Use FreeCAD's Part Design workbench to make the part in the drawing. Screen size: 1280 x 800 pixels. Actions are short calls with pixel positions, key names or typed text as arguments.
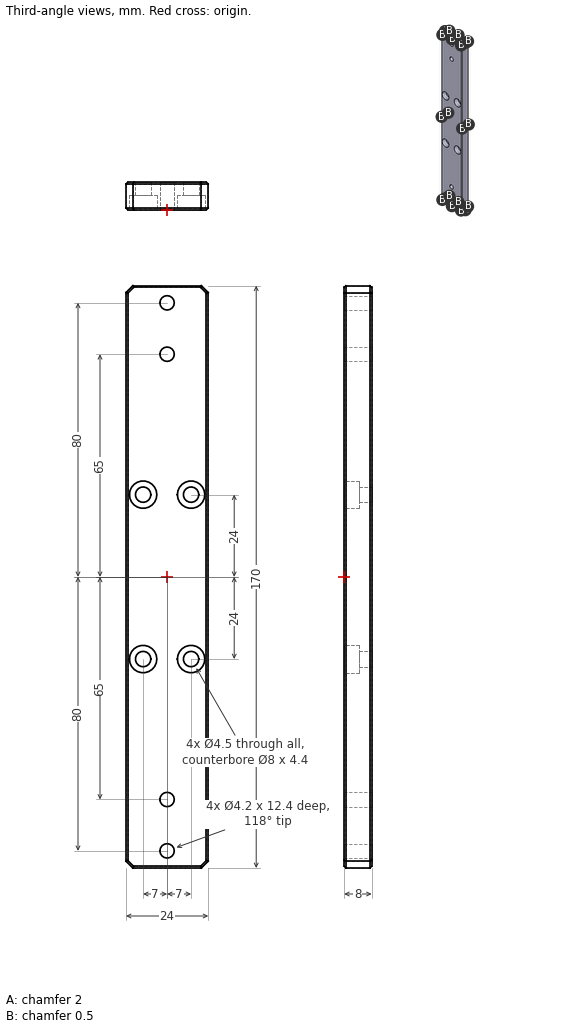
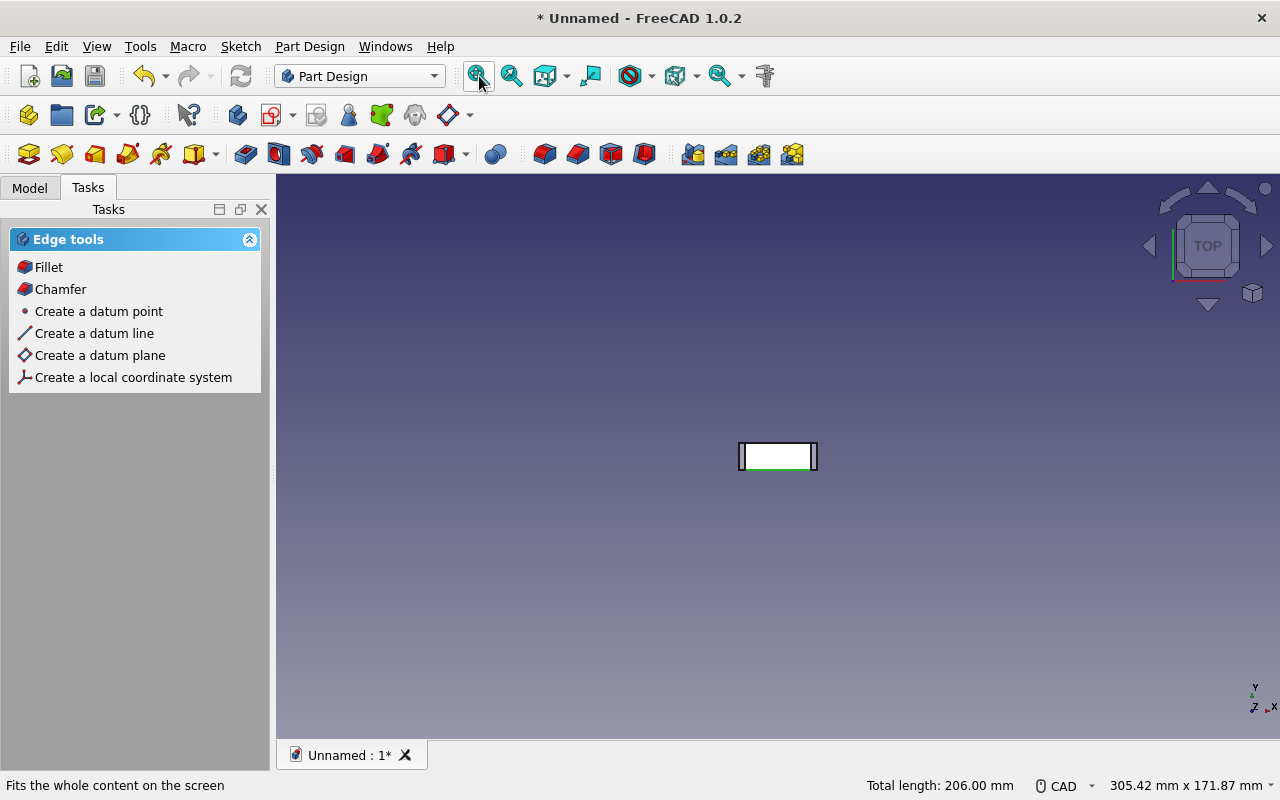
click(778, 442, ctrl)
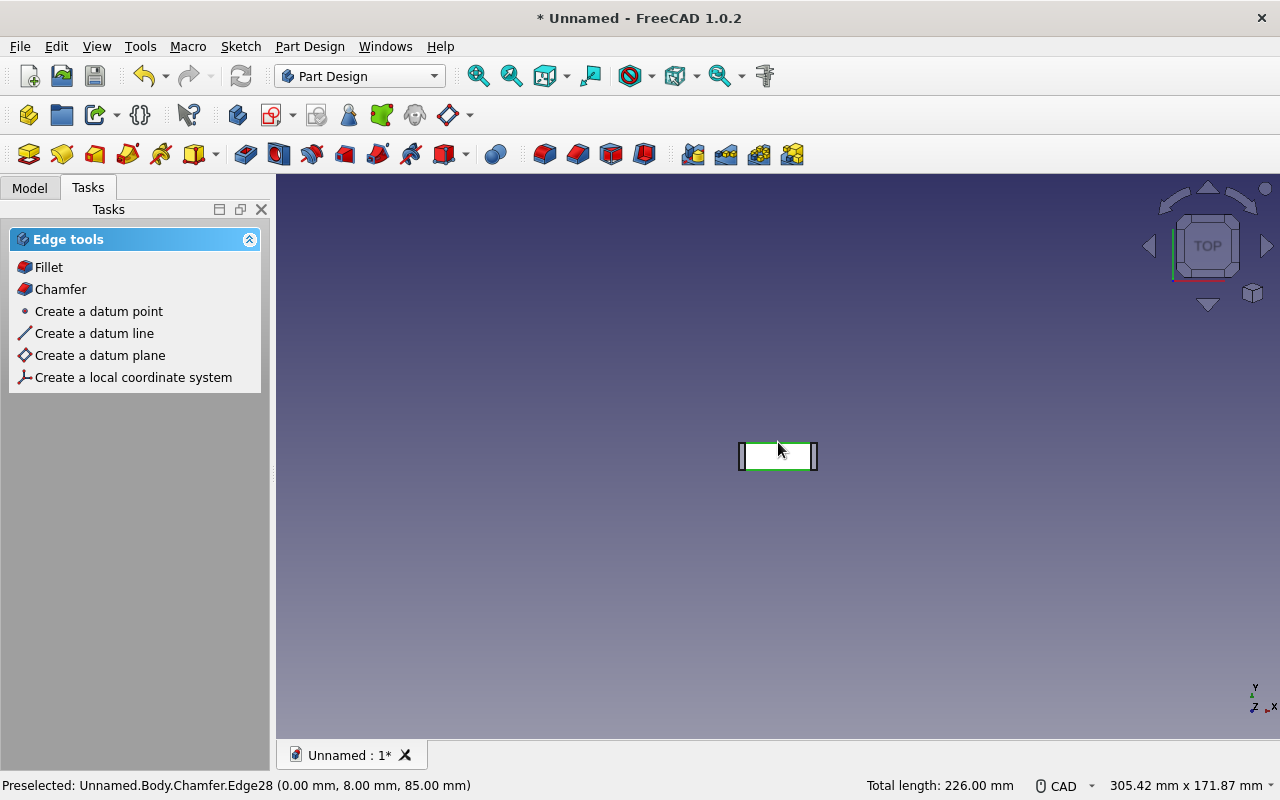
key(1)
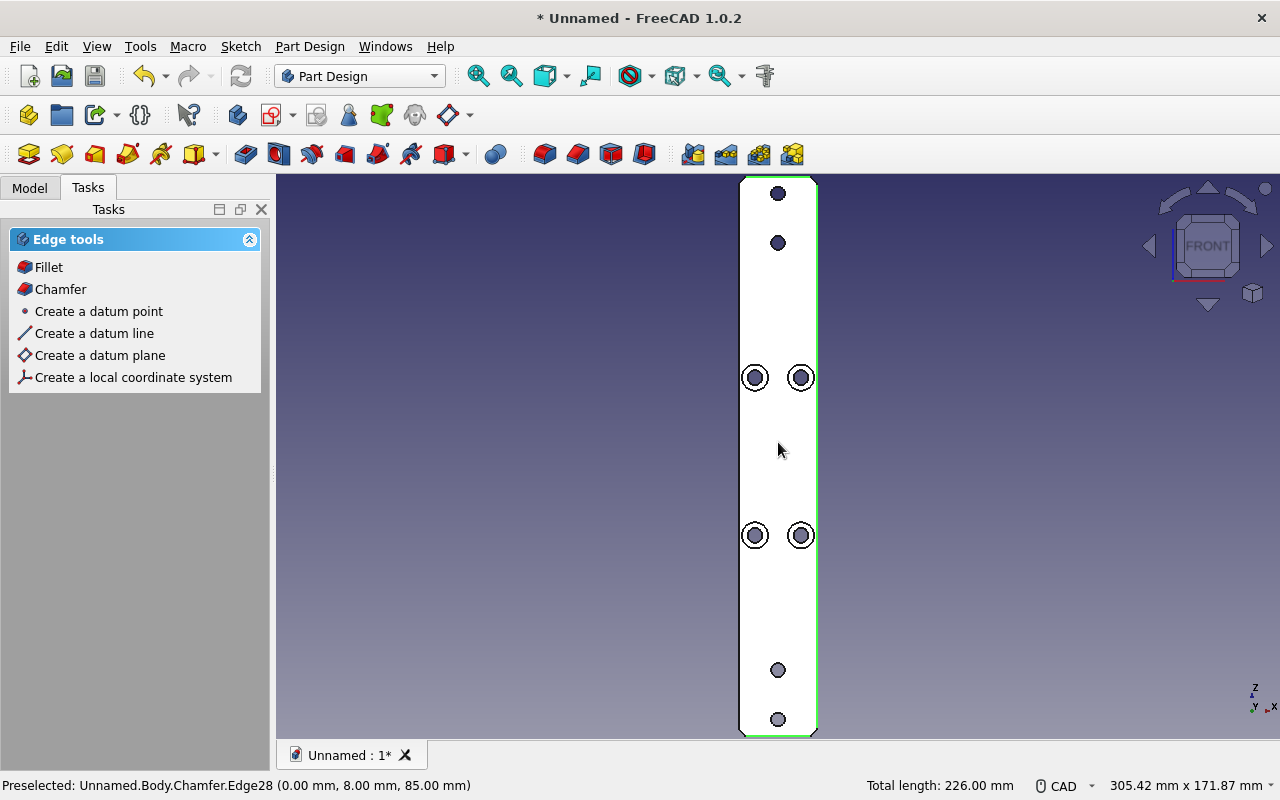
click(739, 456, ctrl)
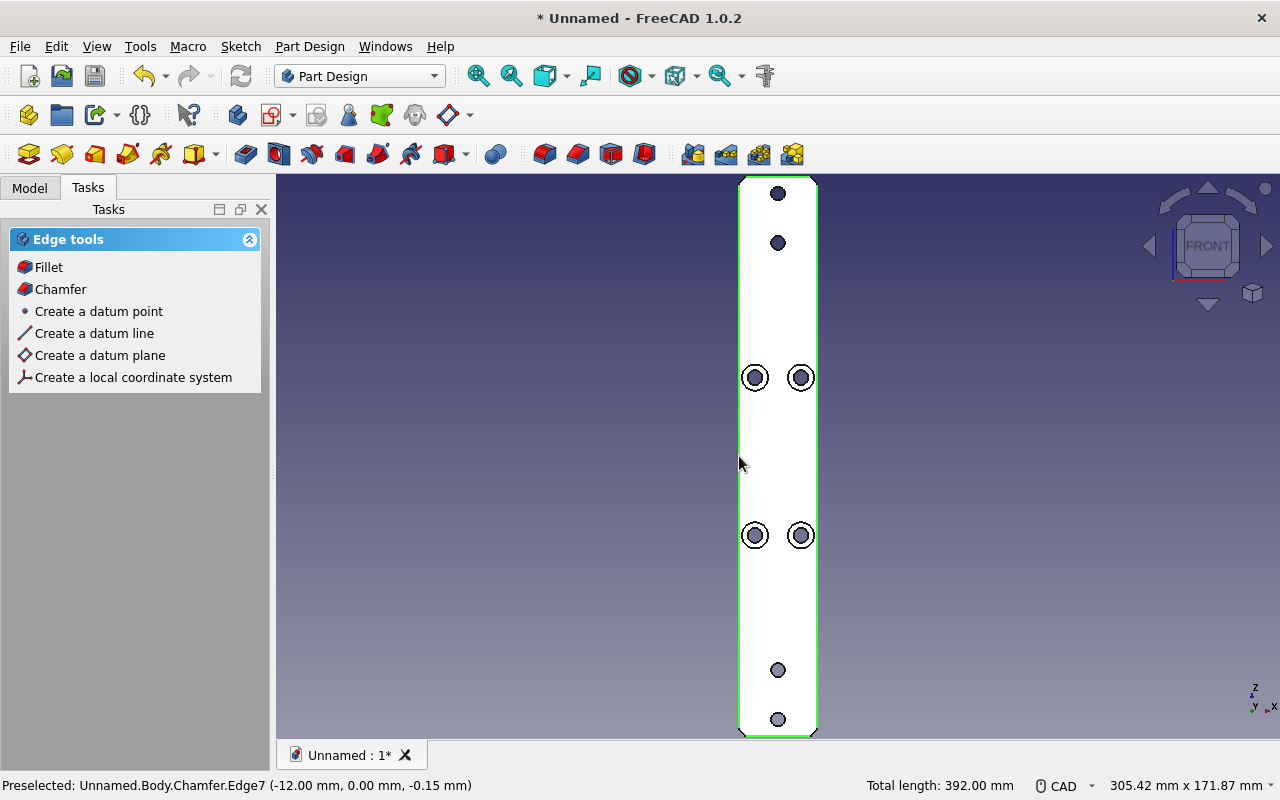
key(3)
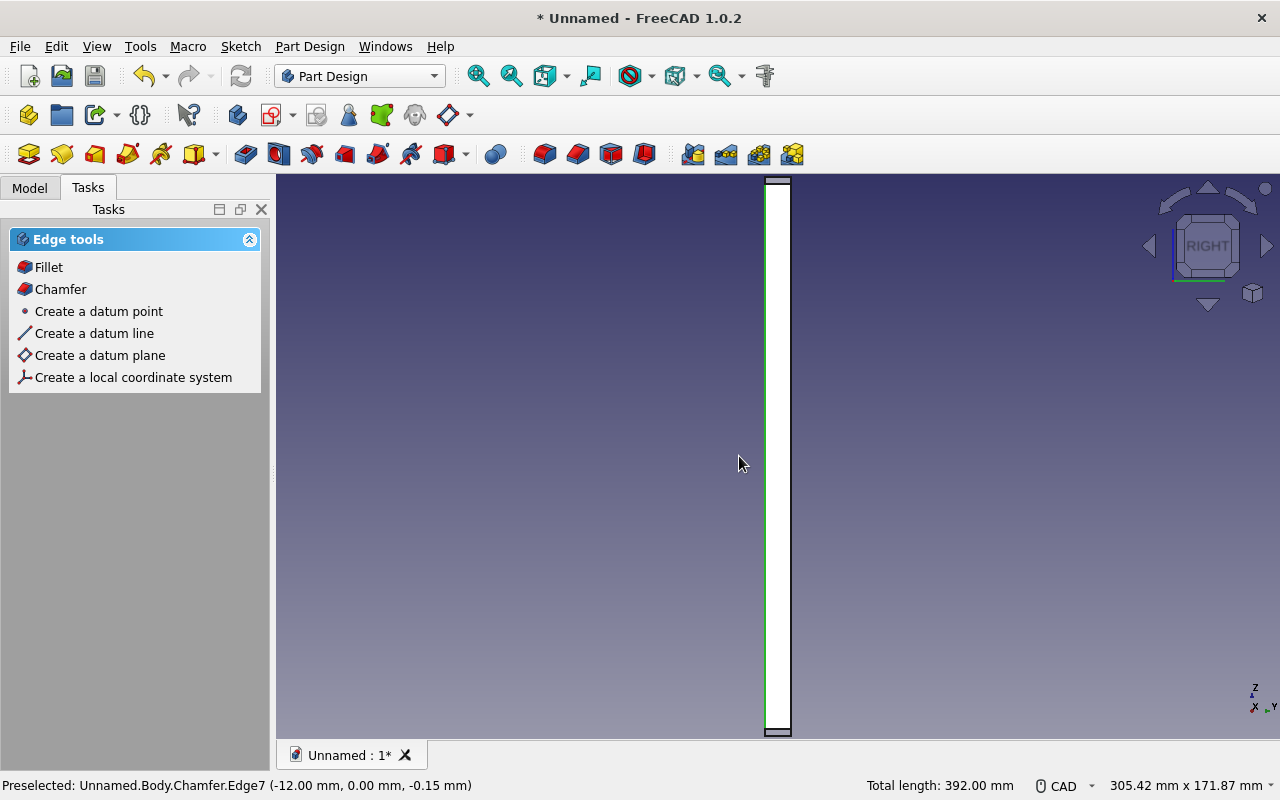
click(791, 455, ctrl)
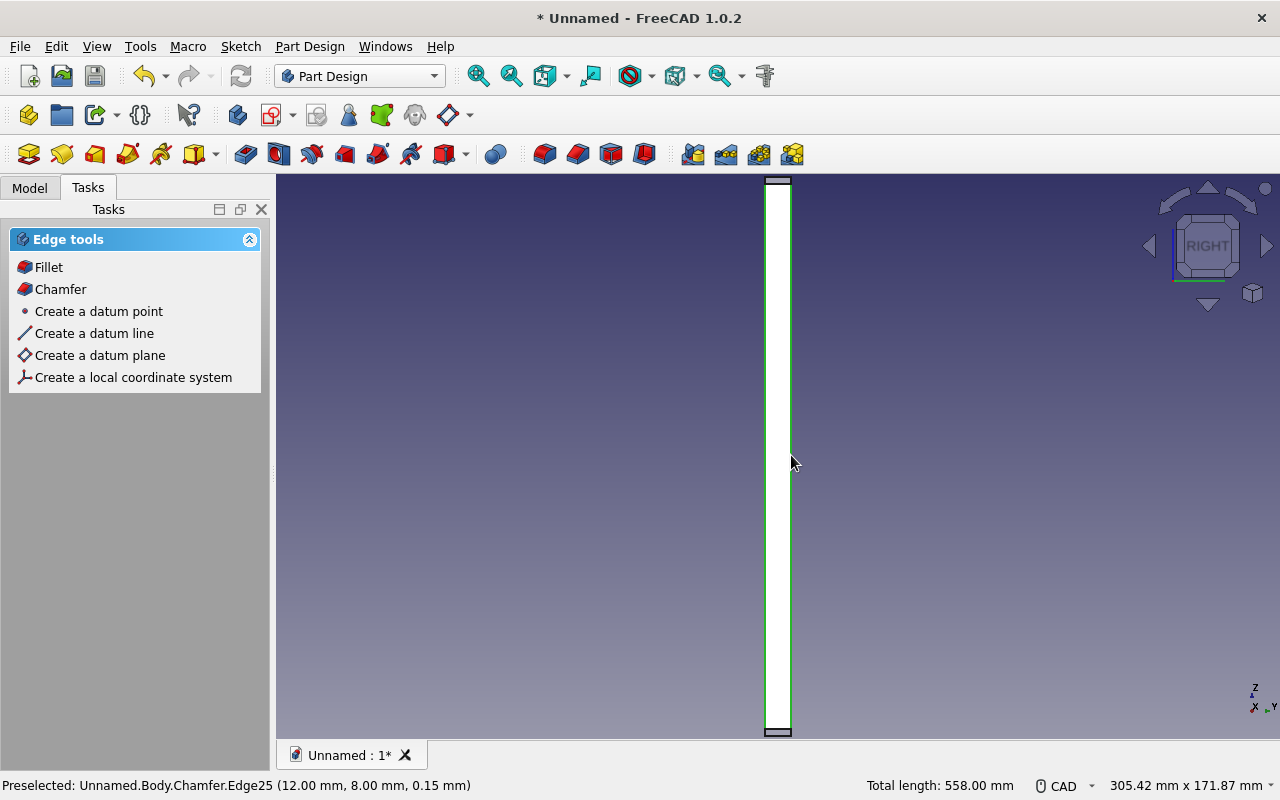
key(5)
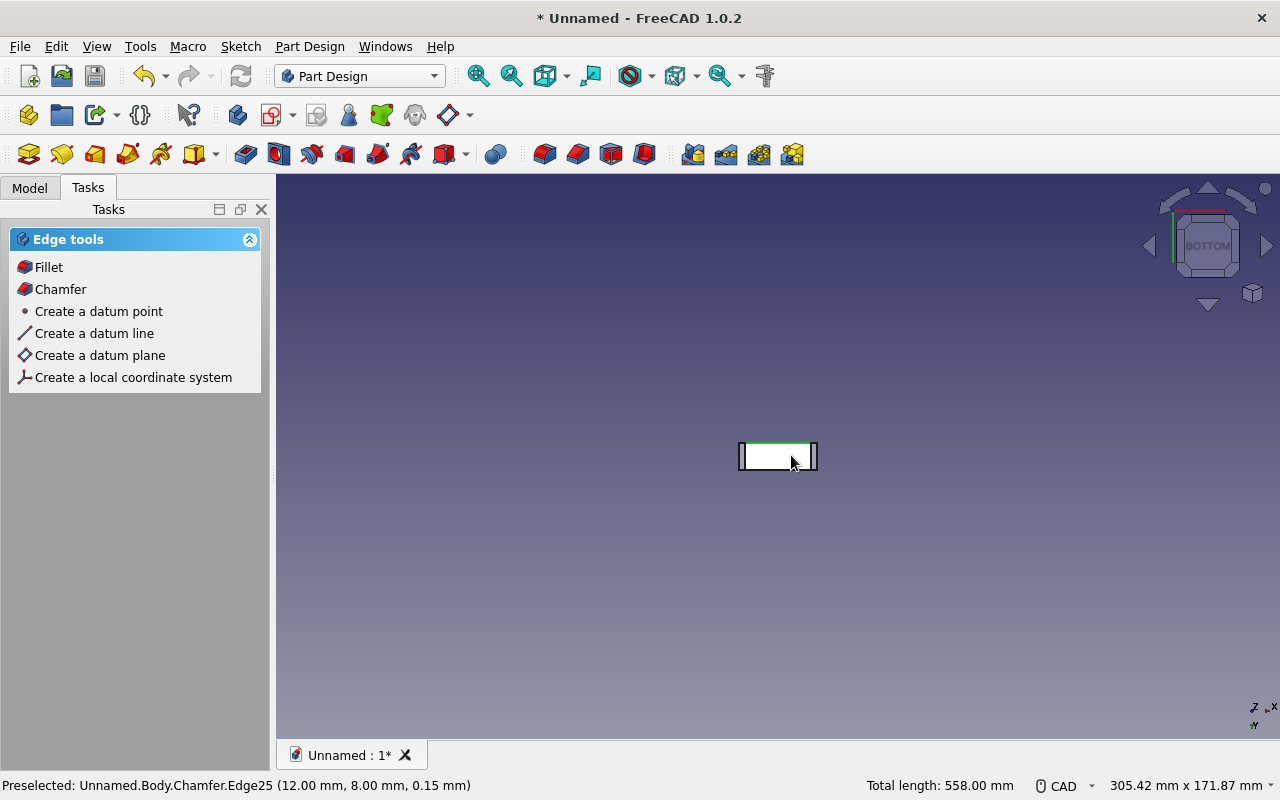
key(v)
key(f)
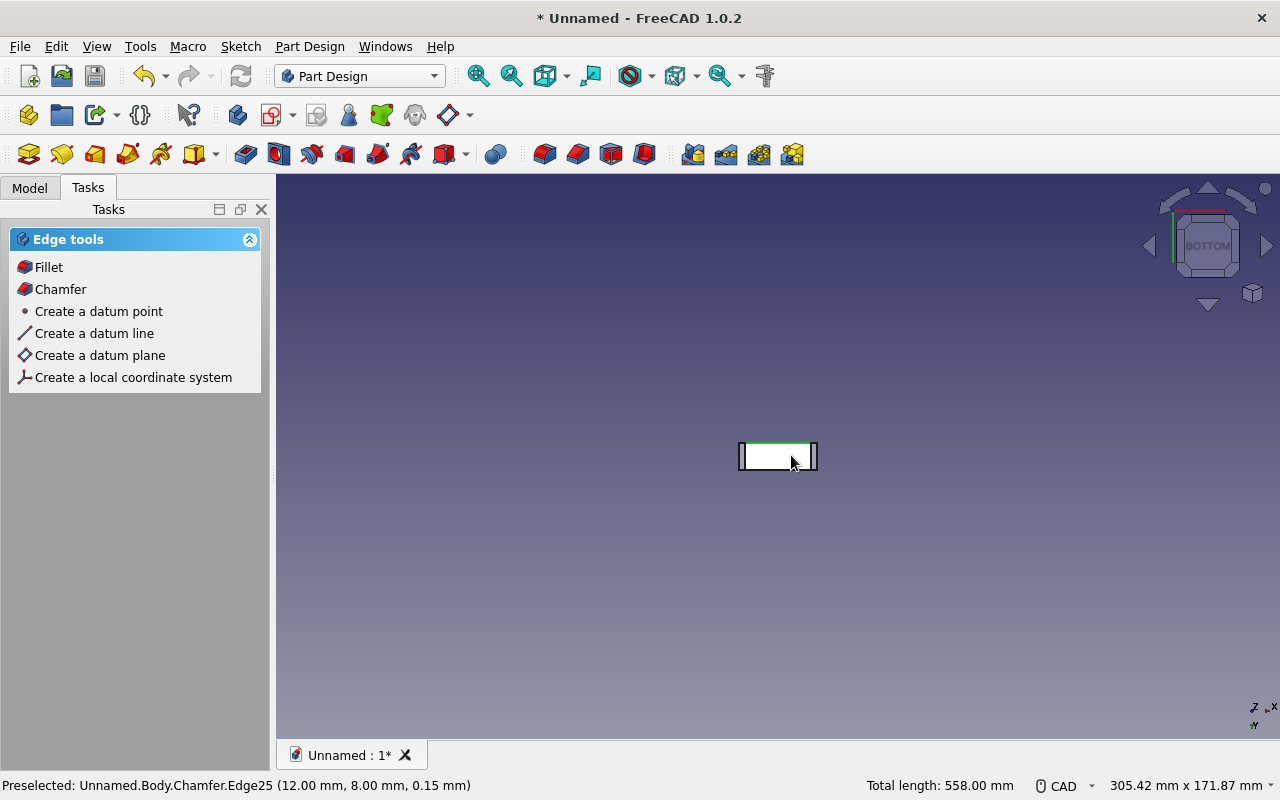
key(4)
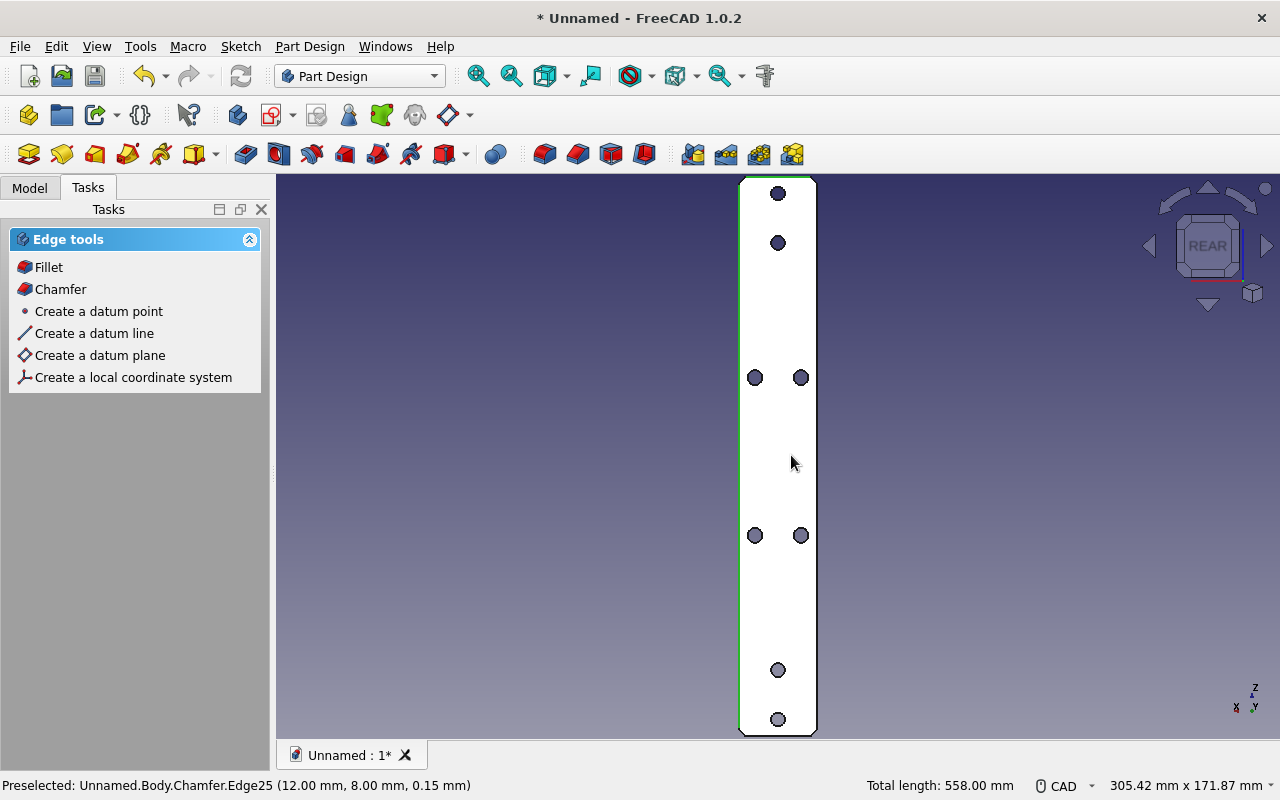
click(817, 456, ctrl)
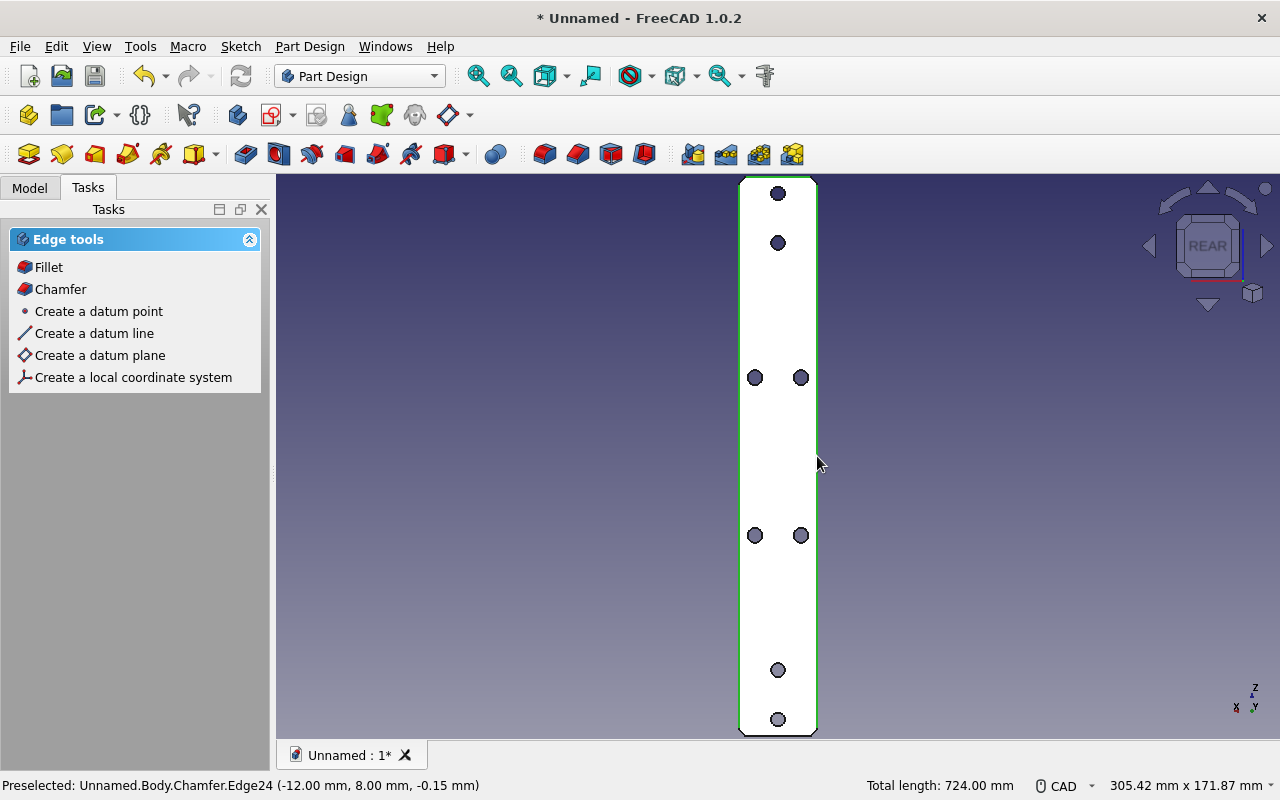
key(6)